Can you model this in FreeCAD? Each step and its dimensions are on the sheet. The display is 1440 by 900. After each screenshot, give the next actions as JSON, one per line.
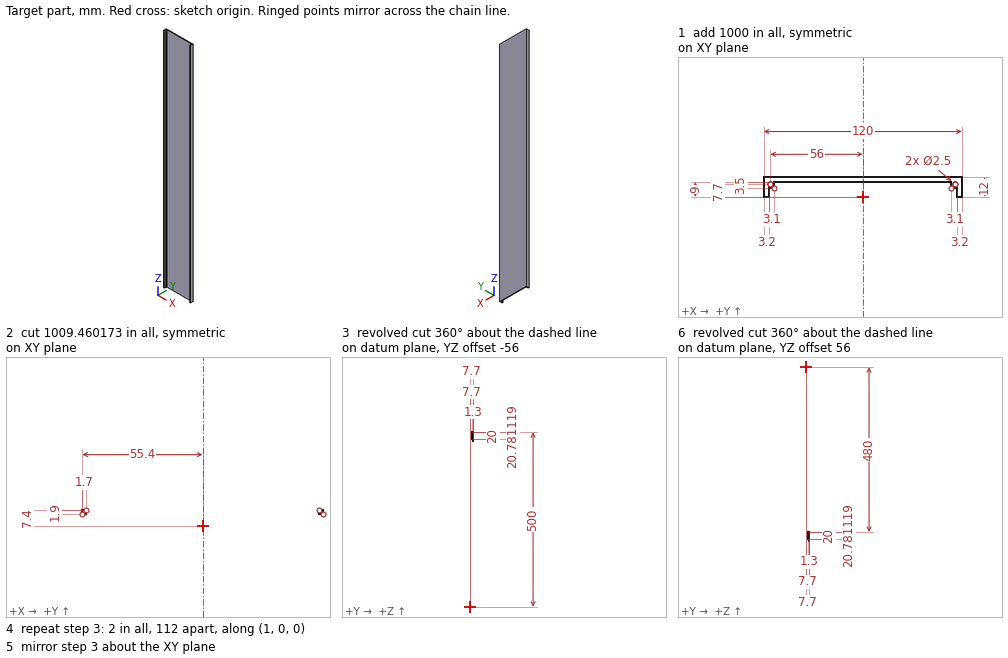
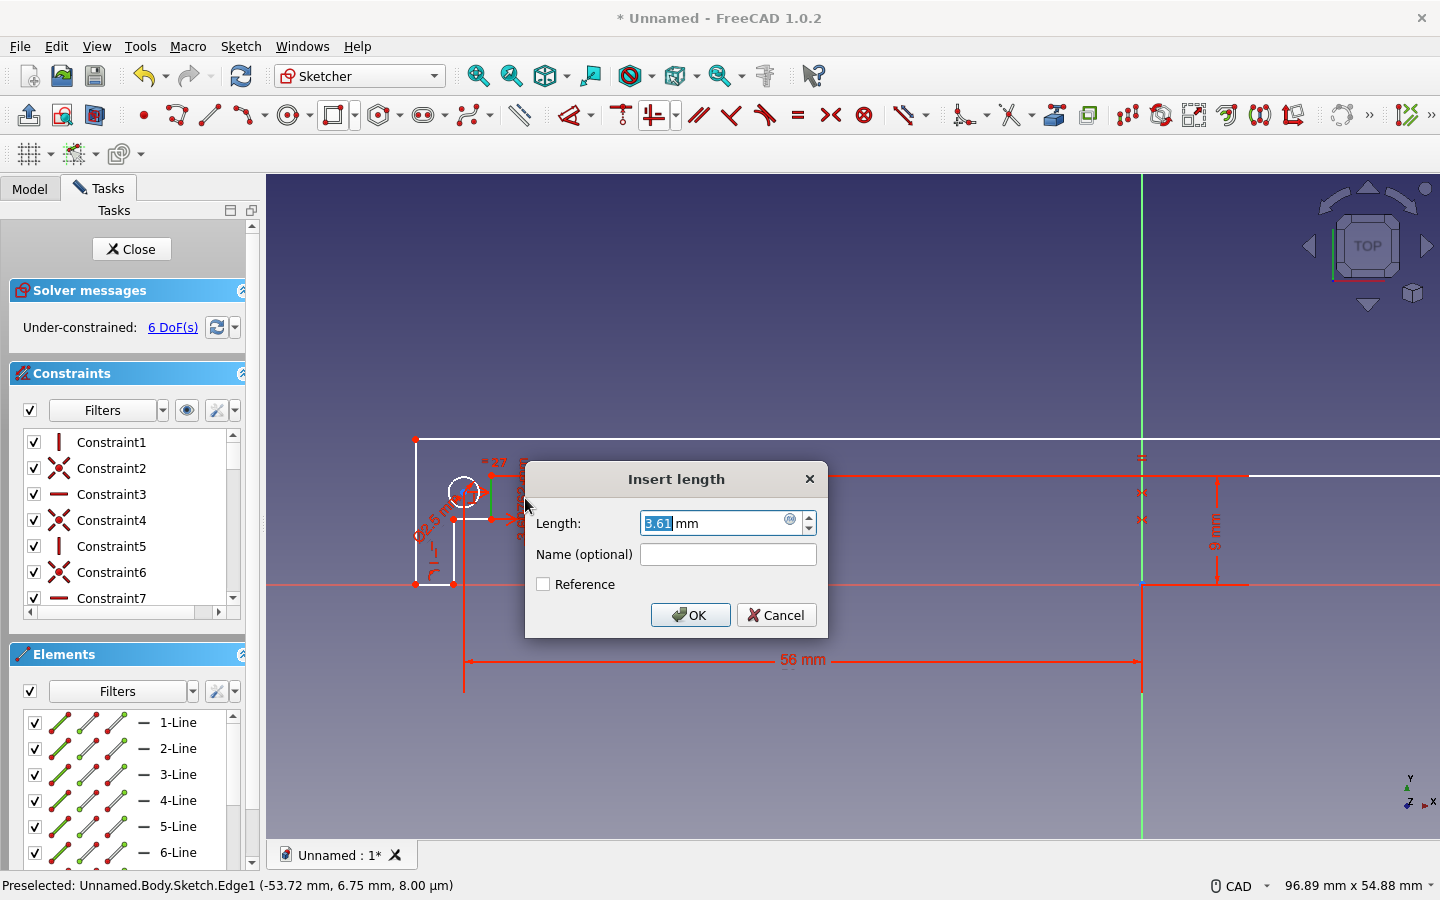
{"action": "type", "text": "3.5"}
{"action": "key", "text": "Return"}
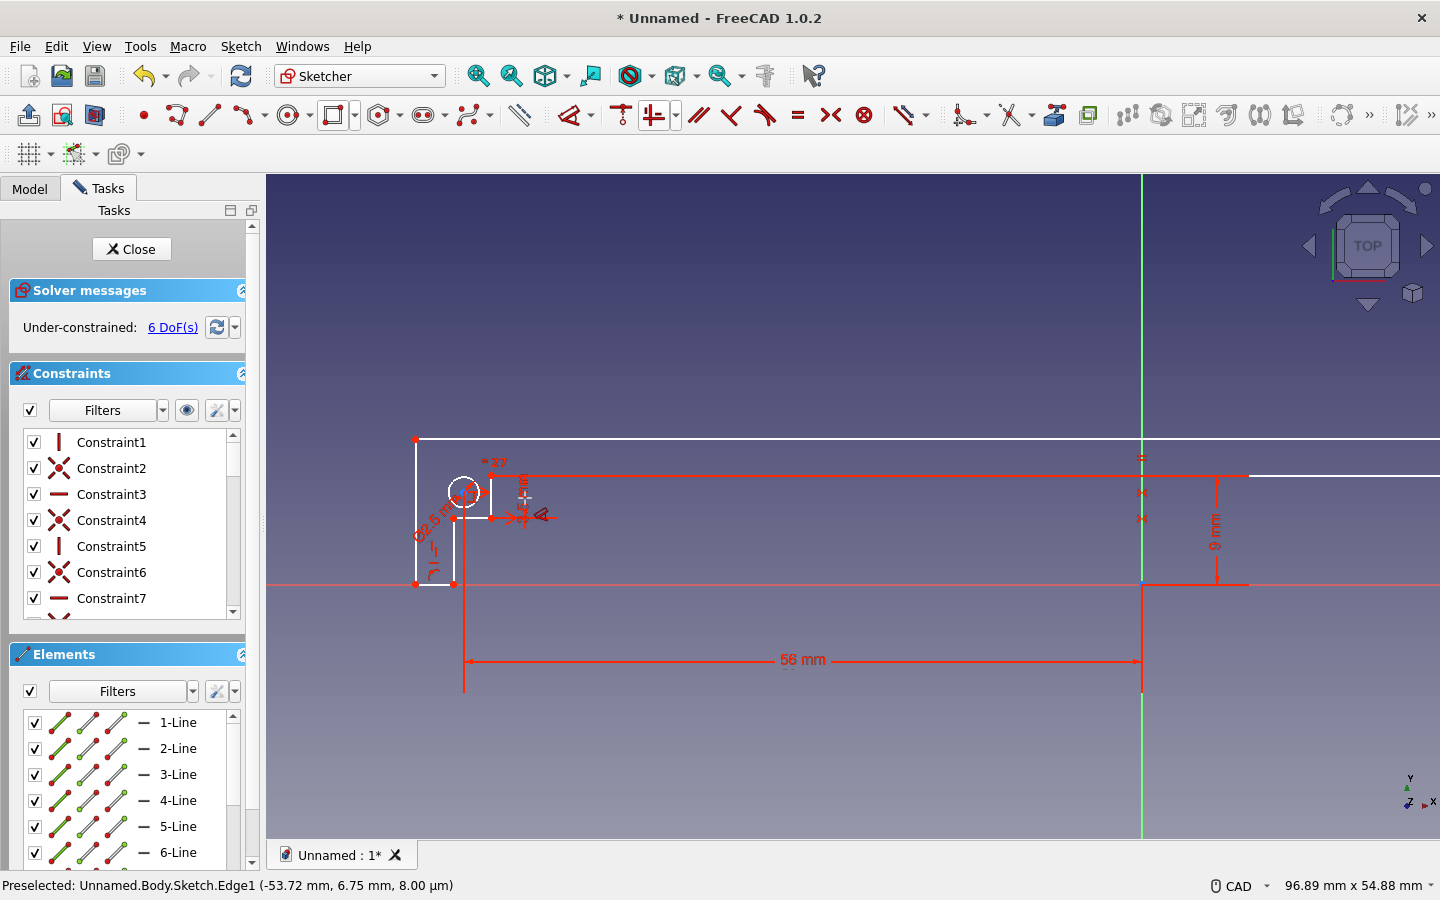
{"action": "scroll", "coordinate": [493, 502], "scroll_direction": "down", "scroll_amount": 4}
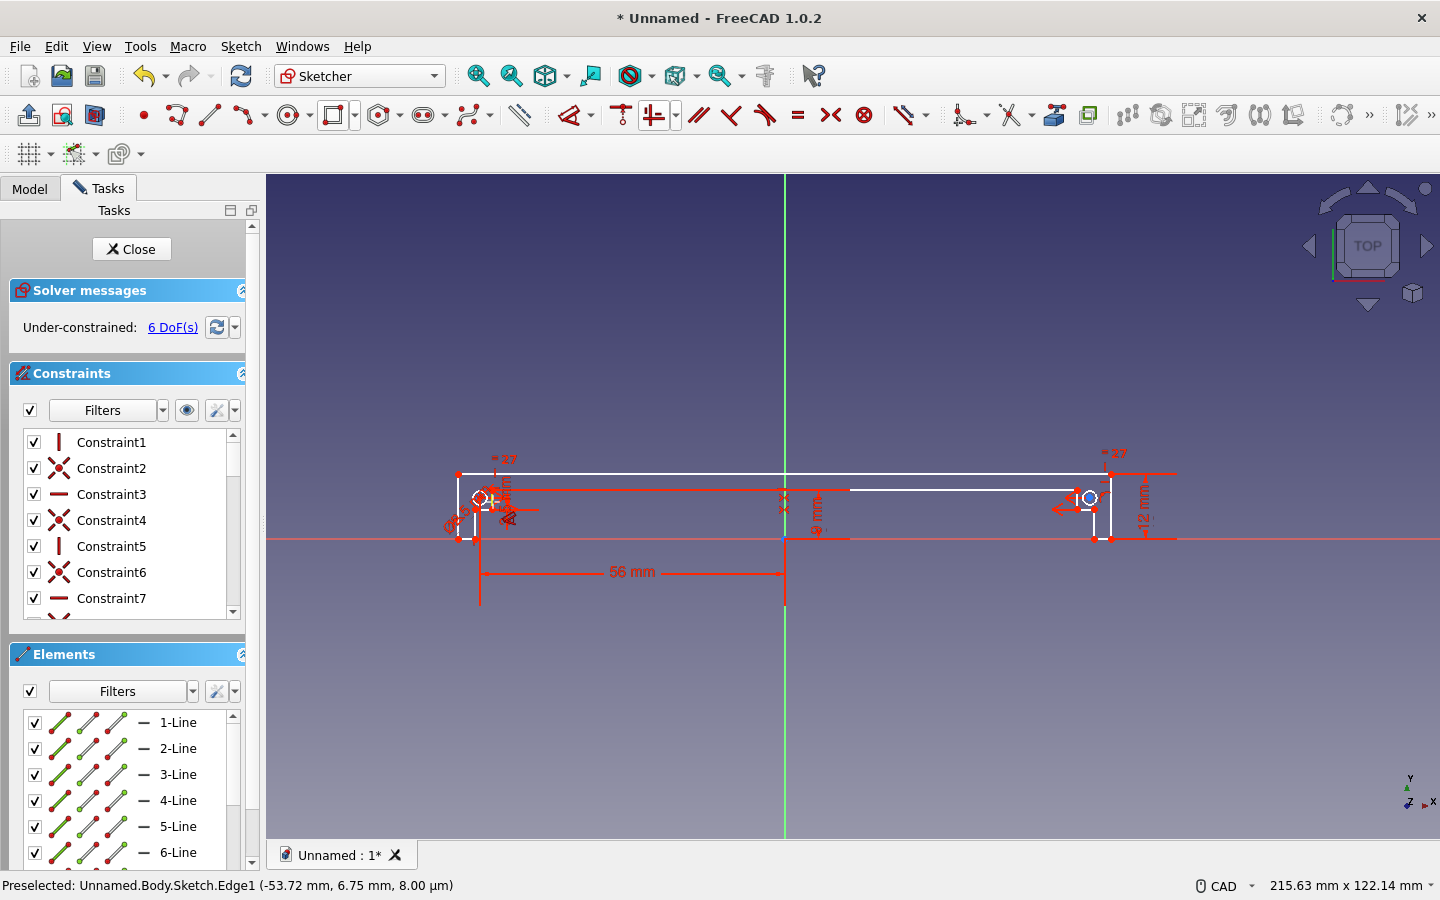
{"action": "scroll", "coordinate": [1082, 510], "scroll_direction": "up", "scroll_amount": 5}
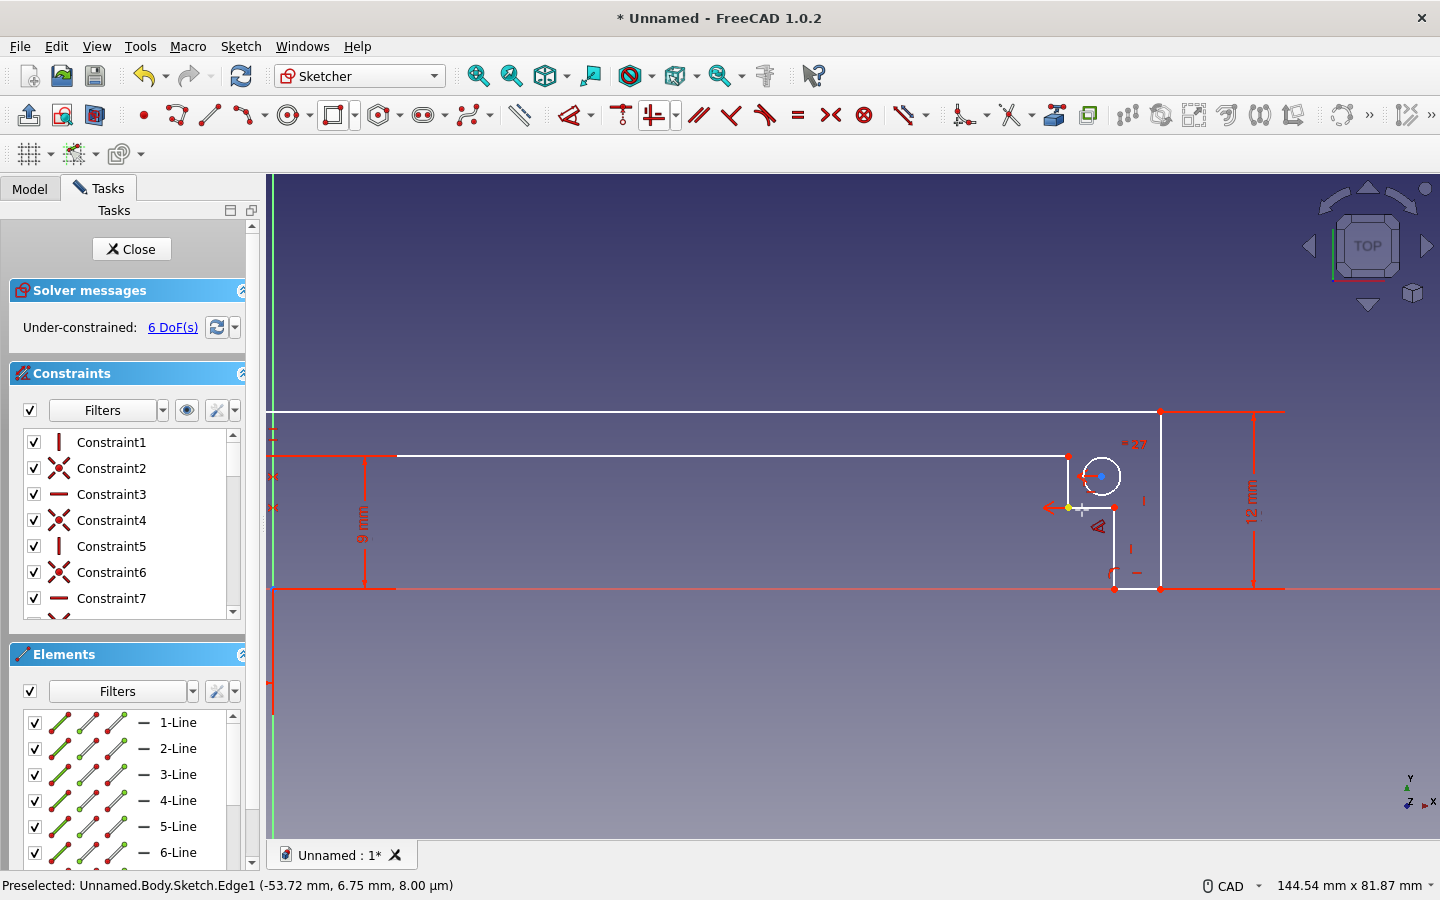
{"action": "left_click", "coordinate": [1082, 508]}
{"action": "left_click", "coordinate": [1091, 542]}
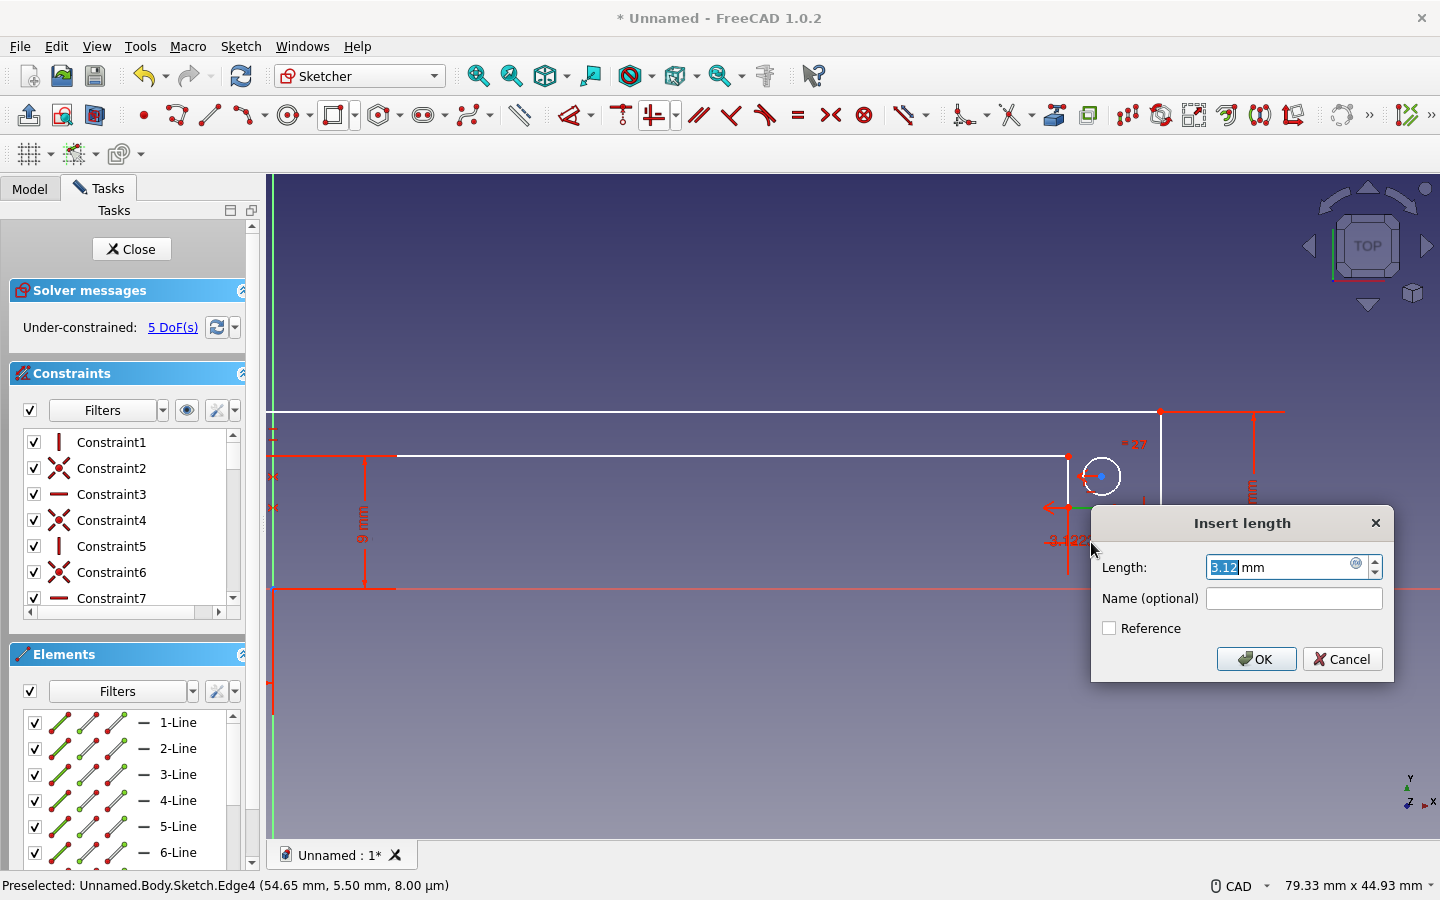
{"action": "type", "text": "3.1"}
{"action": "key", "text": "Return"}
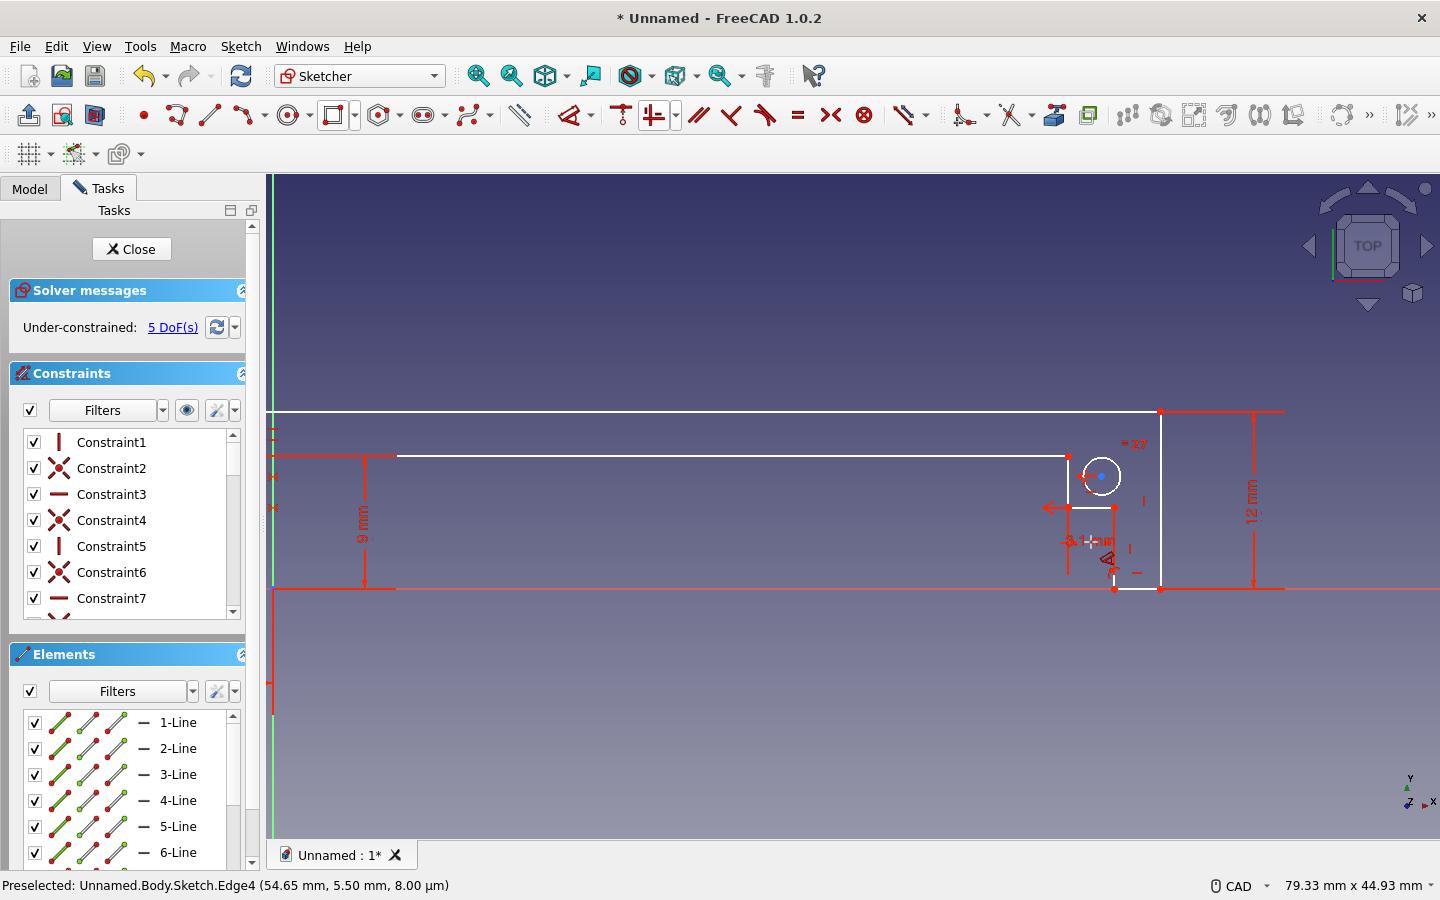
{"action": "left_click", "coordinate": [1128, 589]}
{"action": "left_click", "coordinate": [1137, 623]}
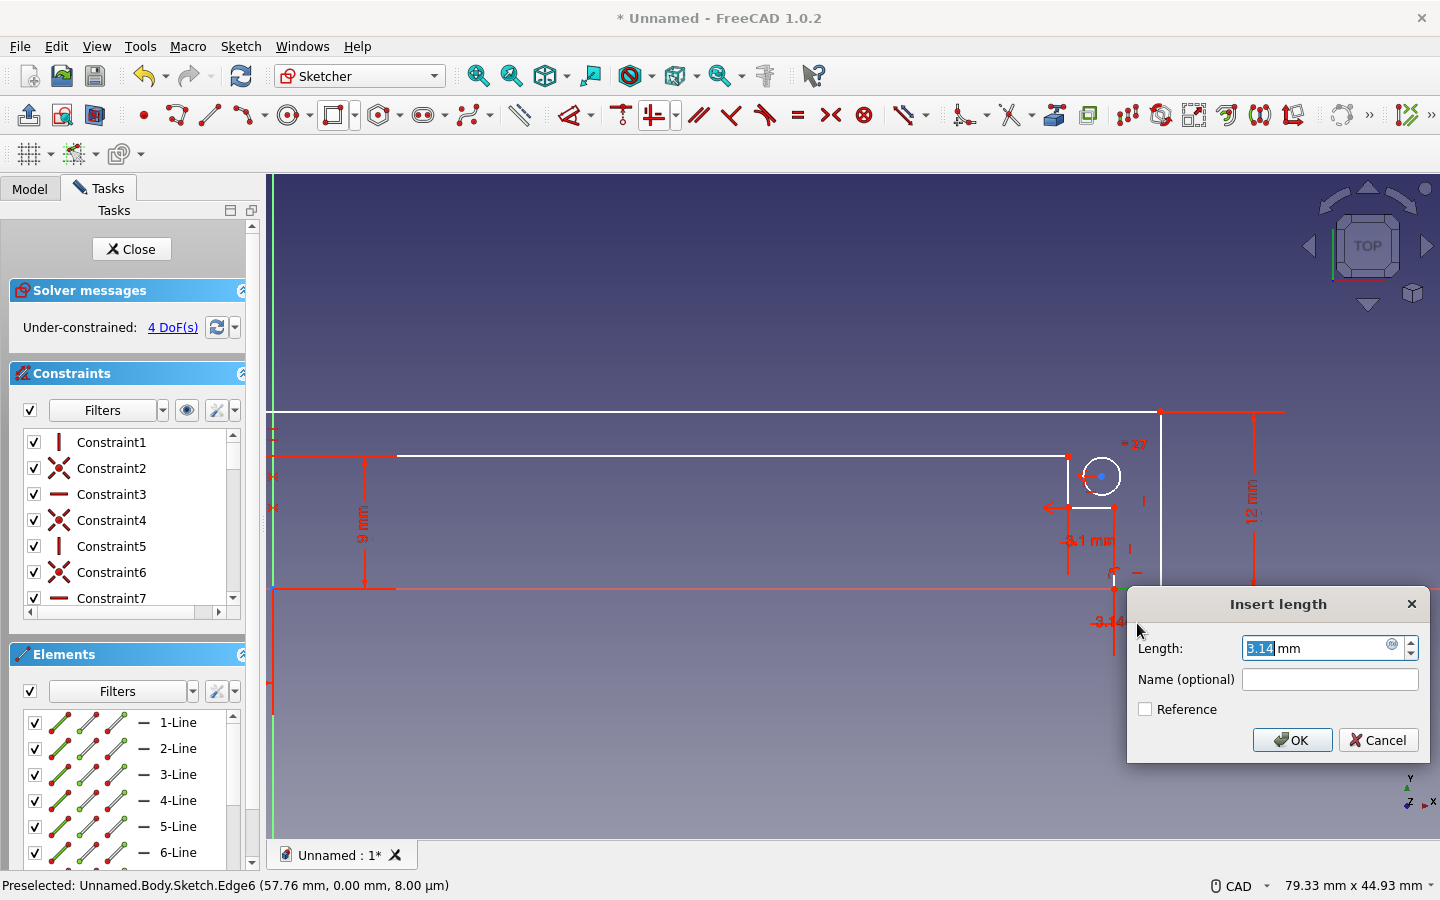
{"action": "type", "text": "3.2"}
{"action": "key", "text": "Return"}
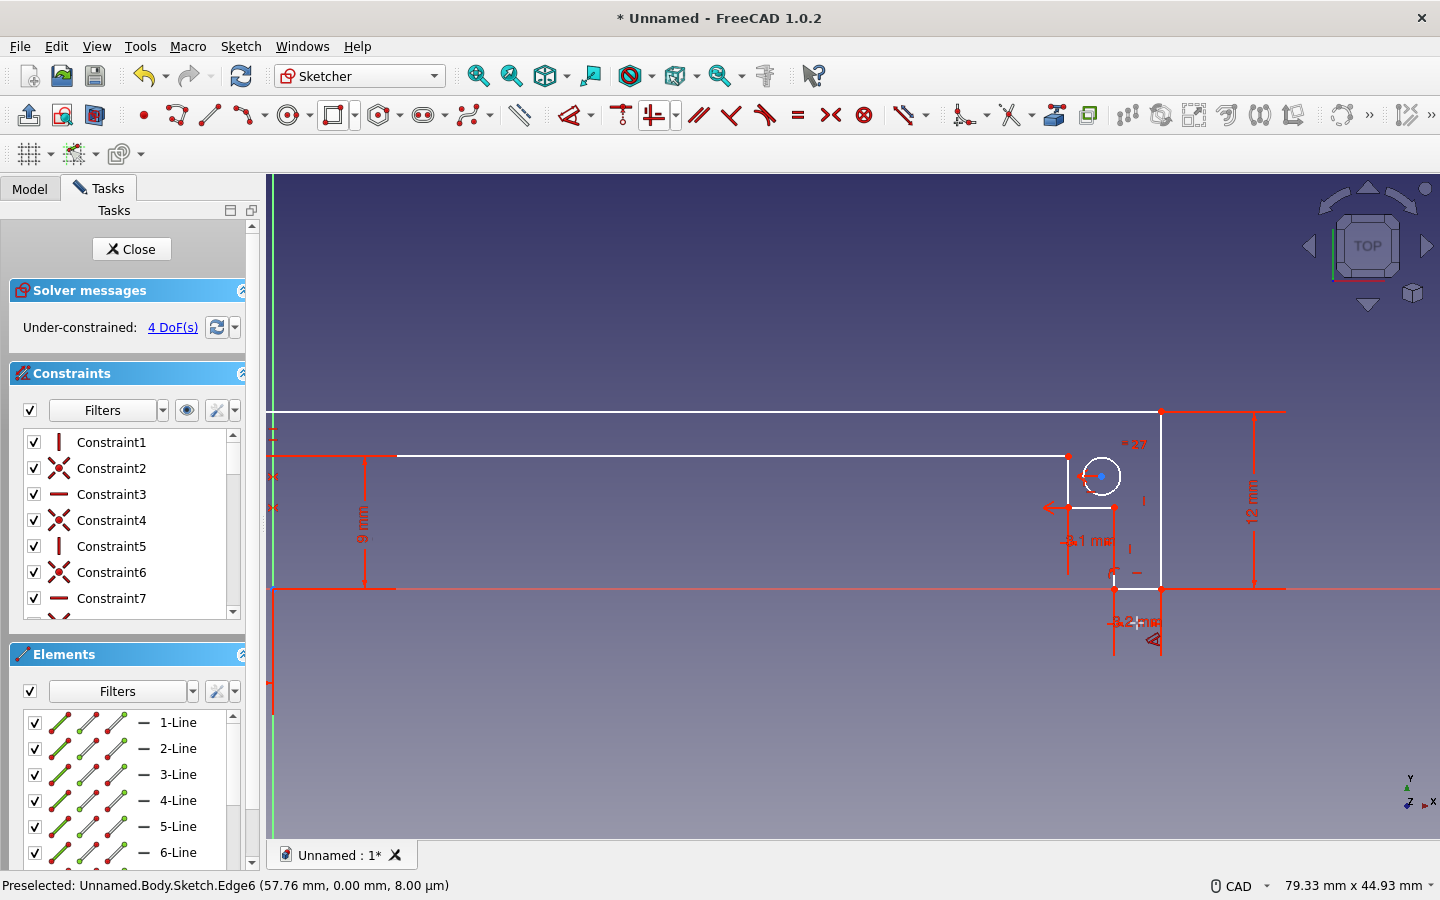
{"action": "left_click", "coordinate": [629, 412]}
{"action": "left_click", "coordinate": [728, 378]}